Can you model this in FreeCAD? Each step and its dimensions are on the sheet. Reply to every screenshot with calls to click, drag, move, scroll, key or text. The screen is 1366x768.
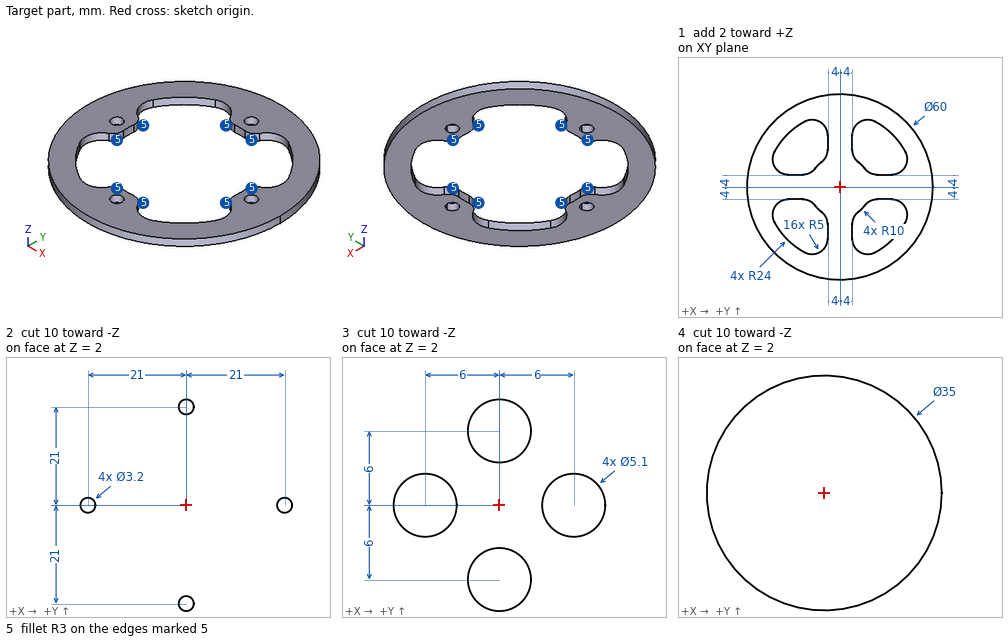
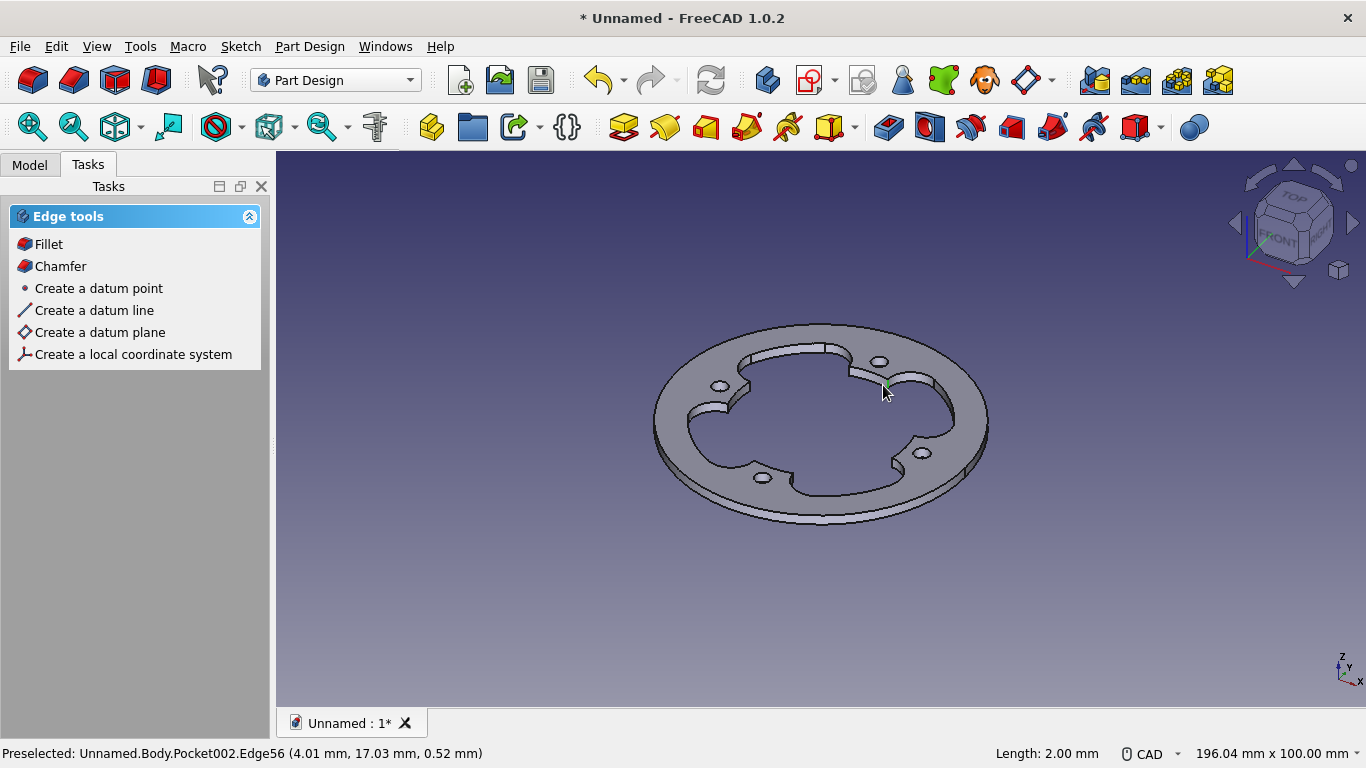
click(728, 409, ctrl)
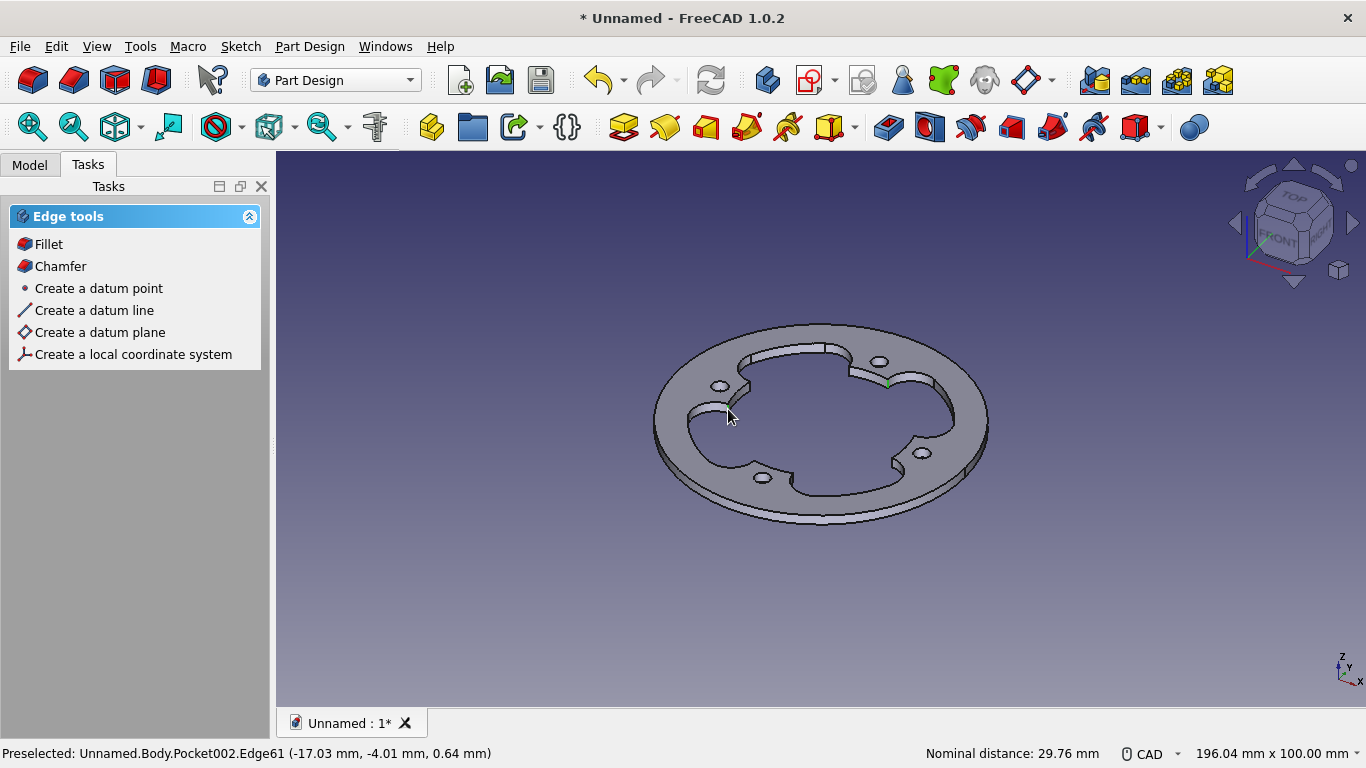
scroll(754, 464, up, 7)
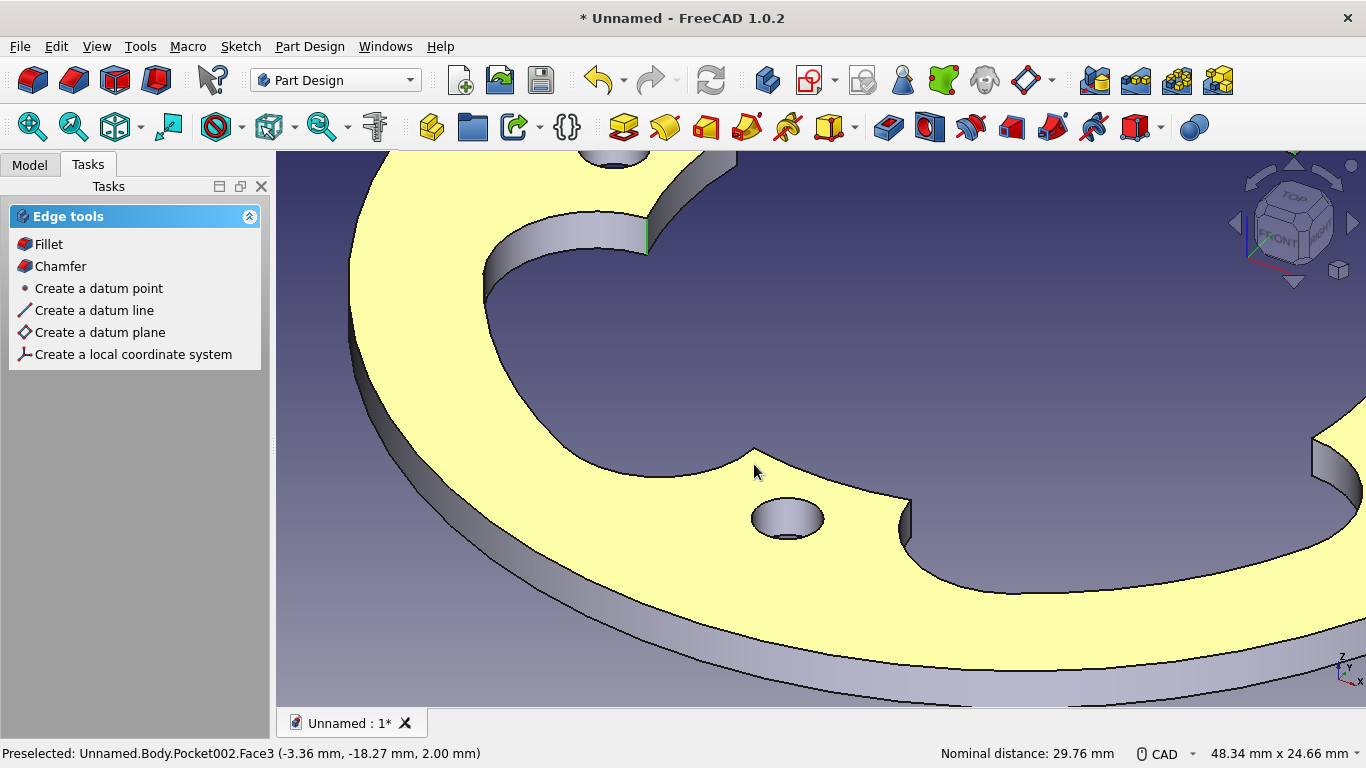
click(33, 128)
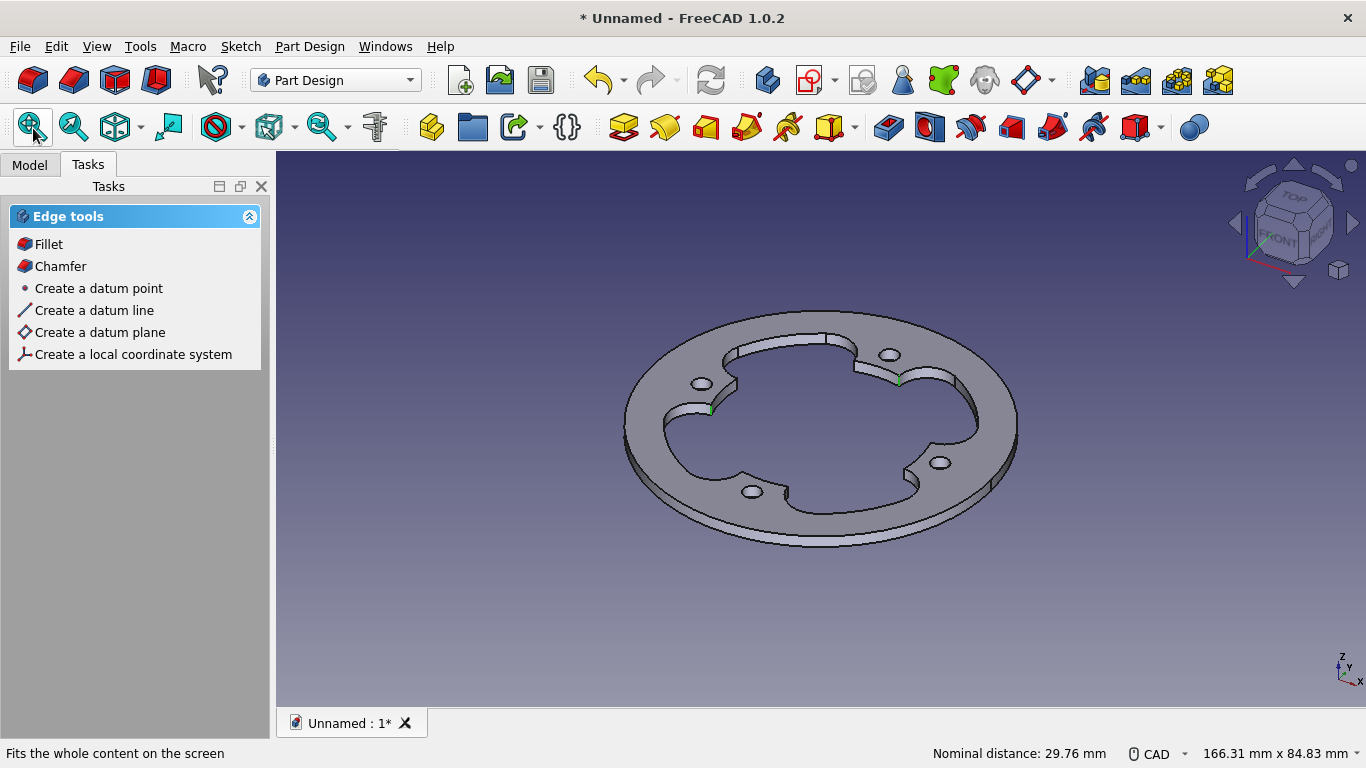
key(0)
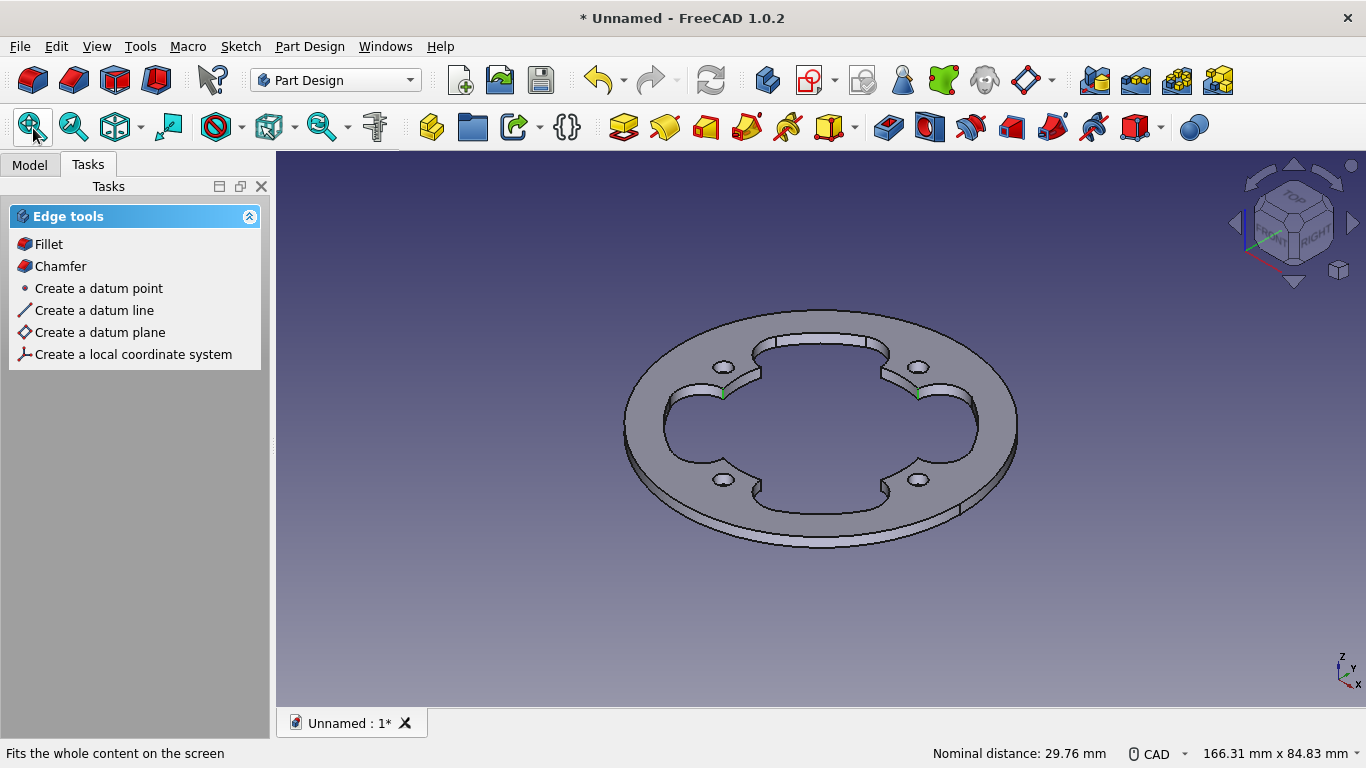
scroll(723, 463, up, 6)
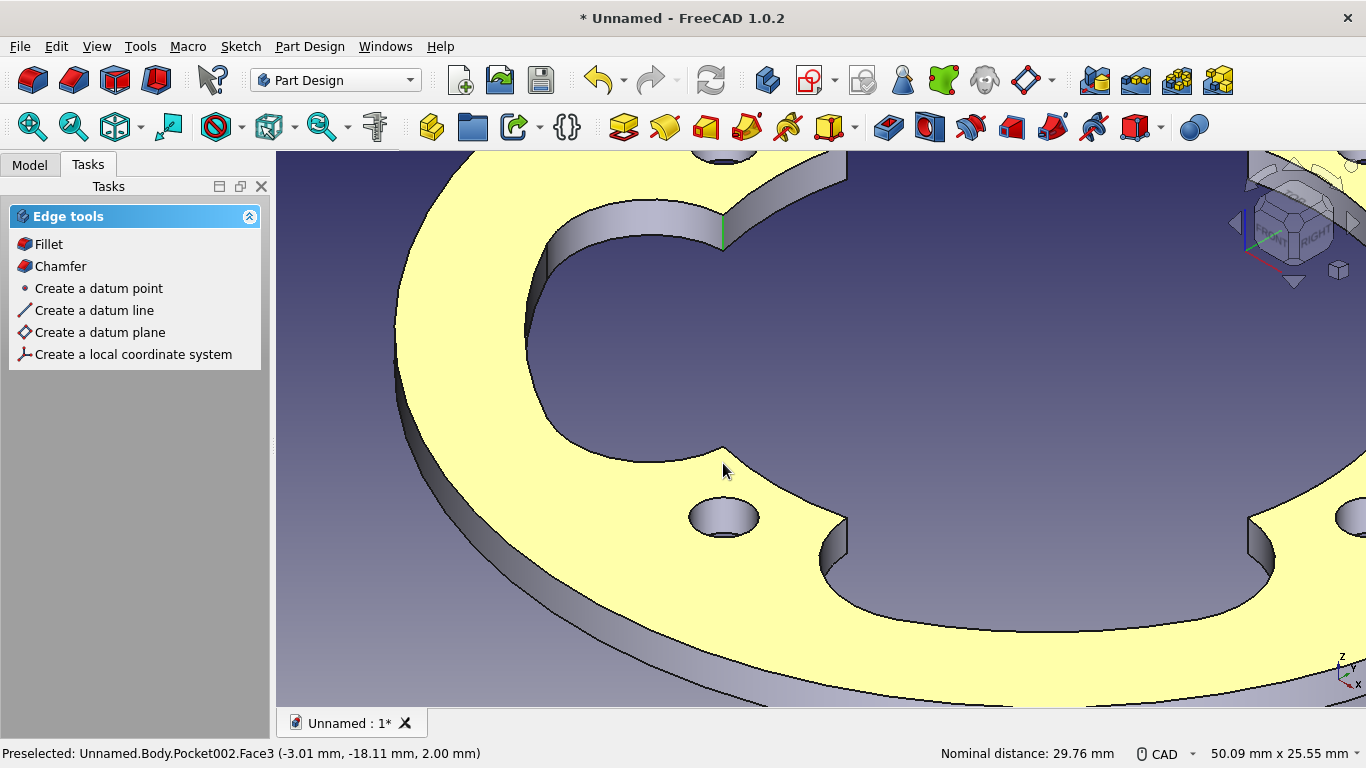
click(33, 128)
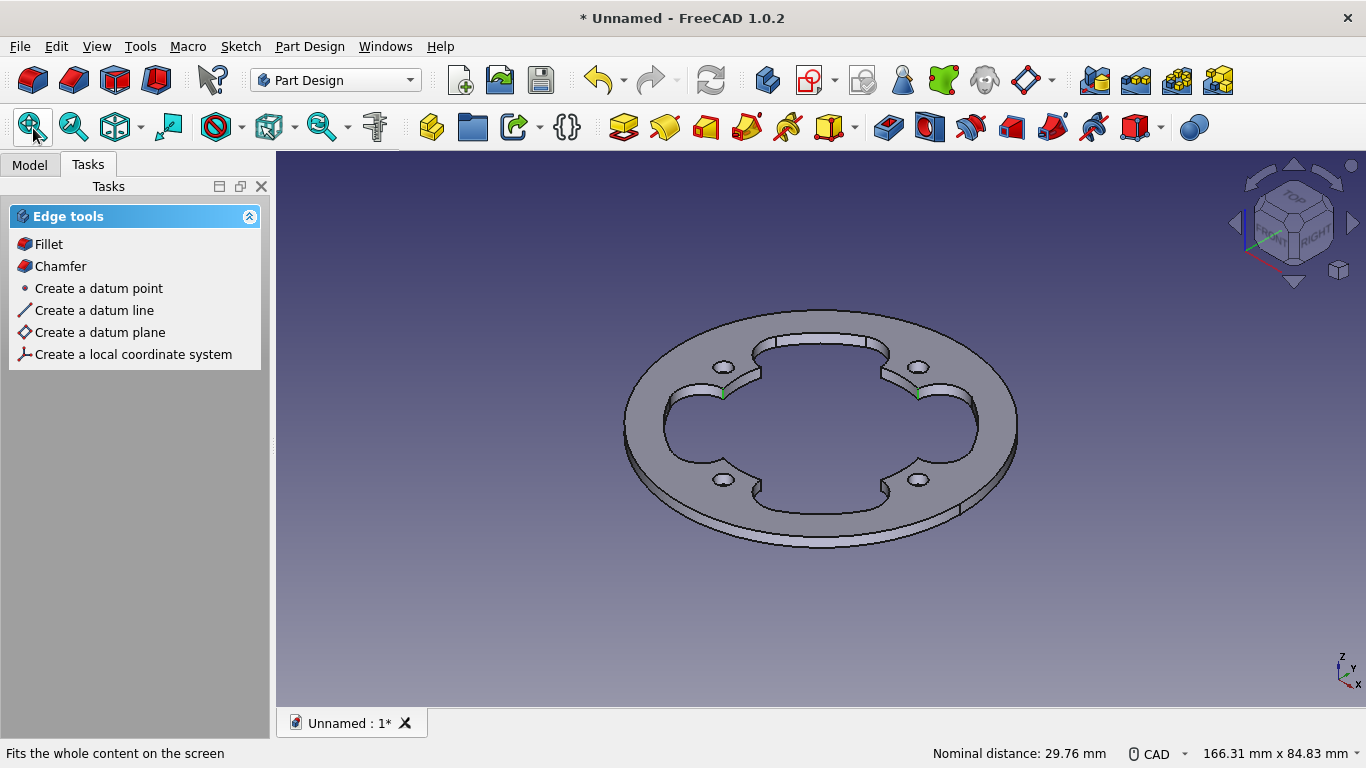
key(2)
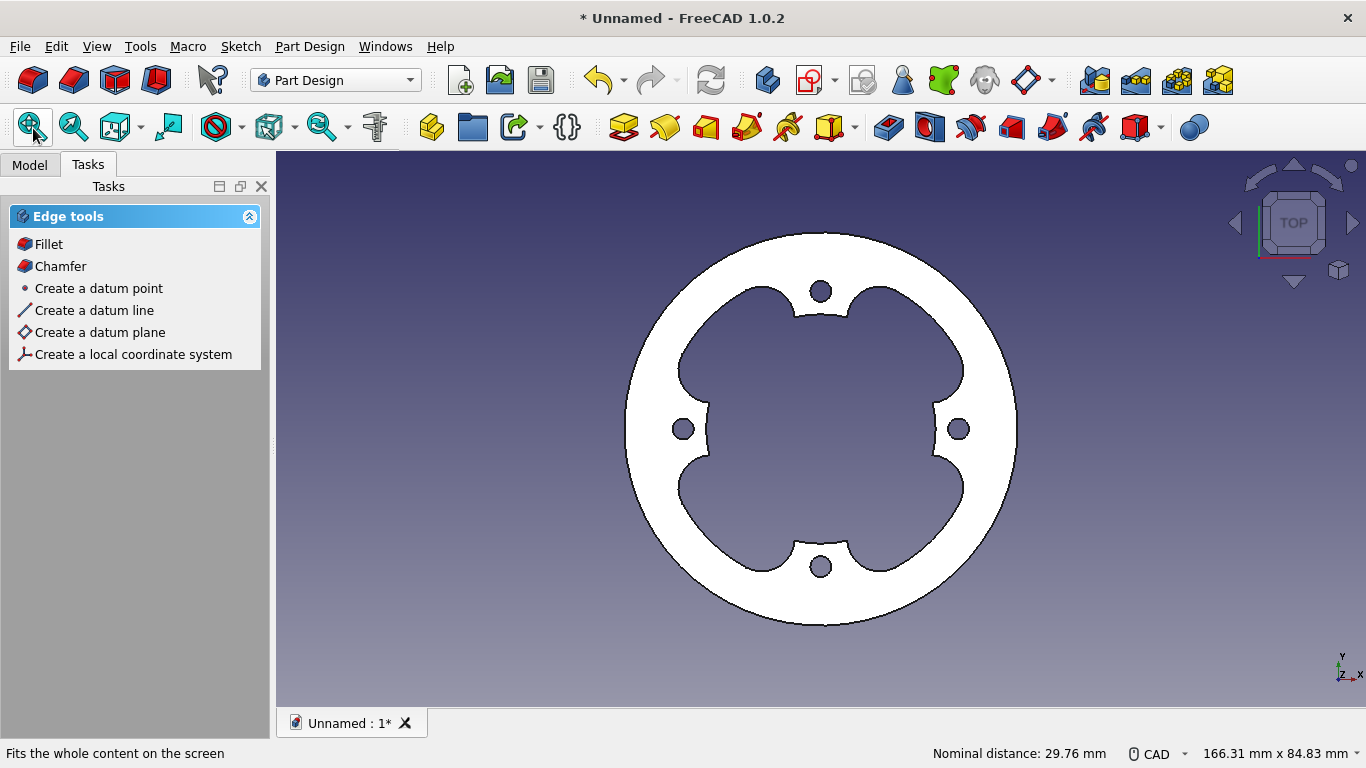
scroll(795, 540, up, 6)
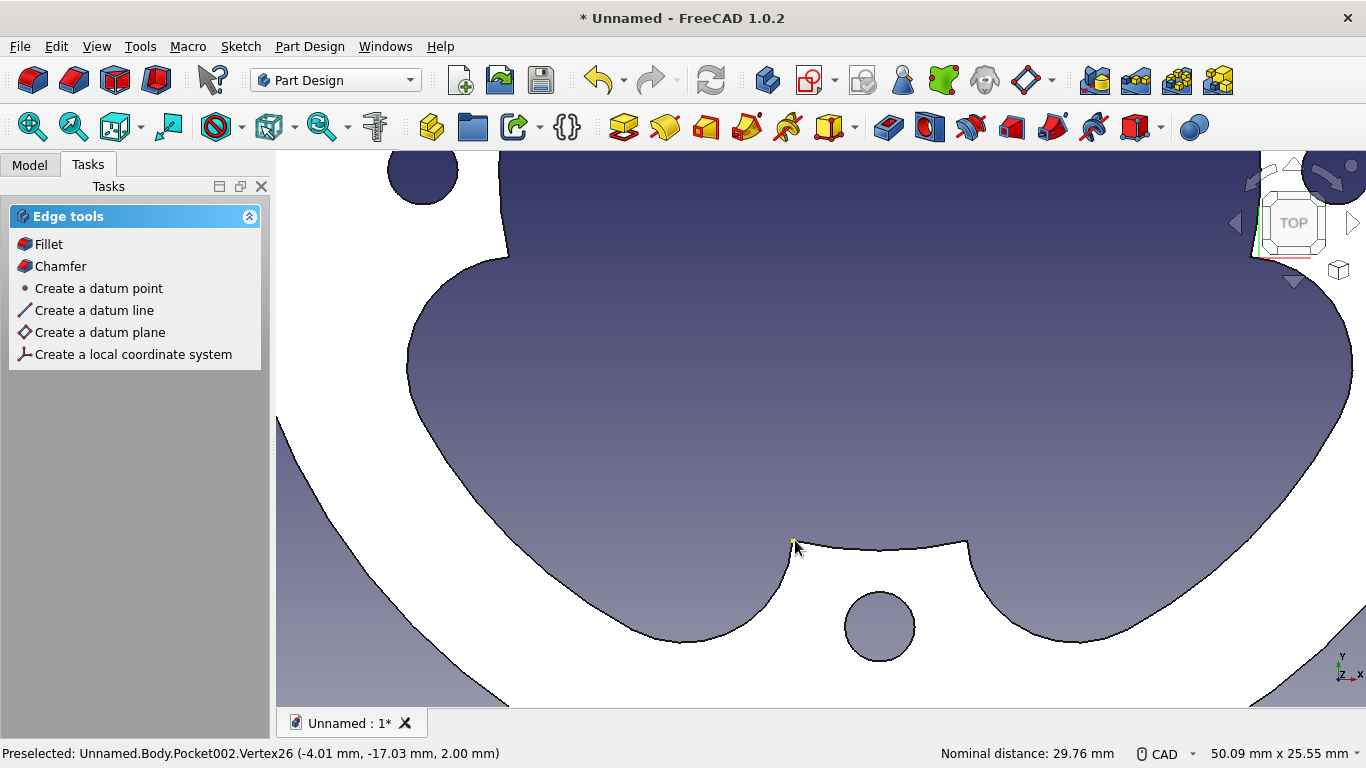
key(v)
key(f)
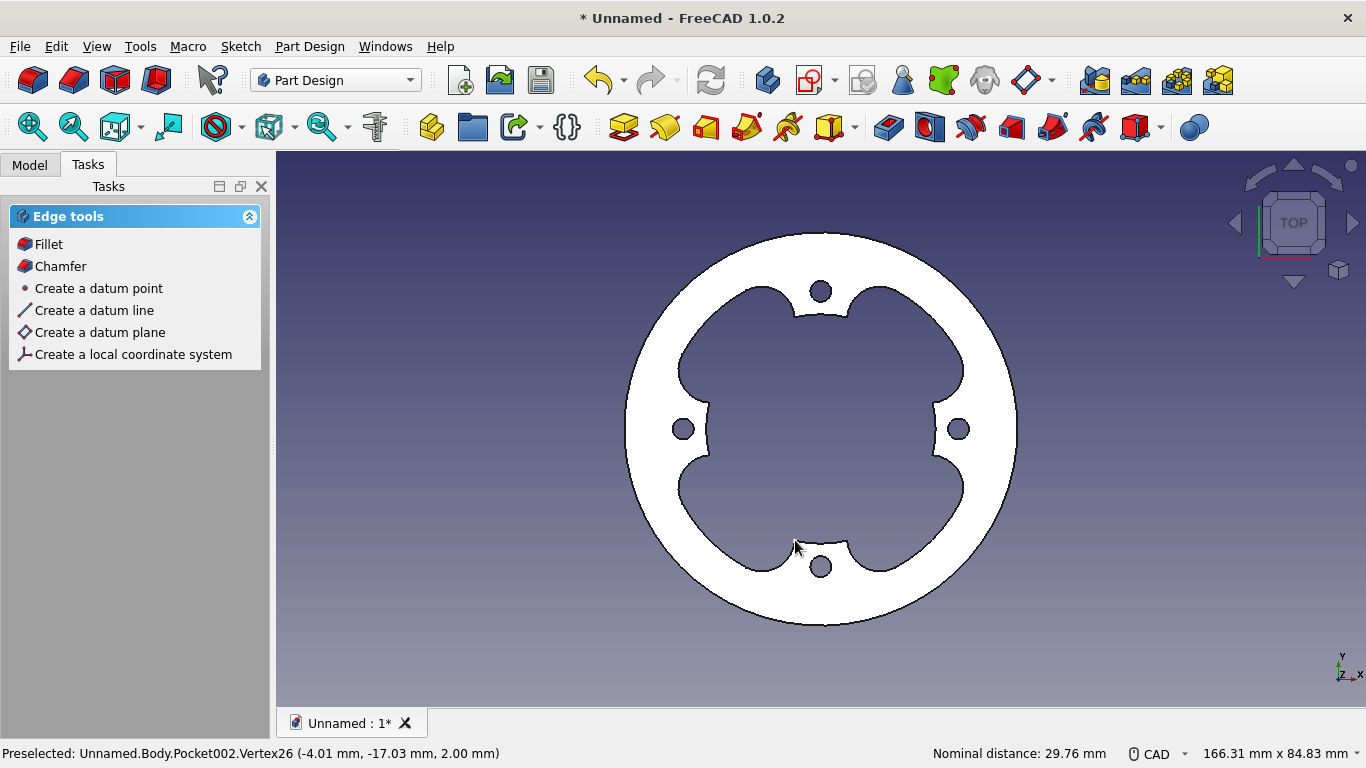
key(1)